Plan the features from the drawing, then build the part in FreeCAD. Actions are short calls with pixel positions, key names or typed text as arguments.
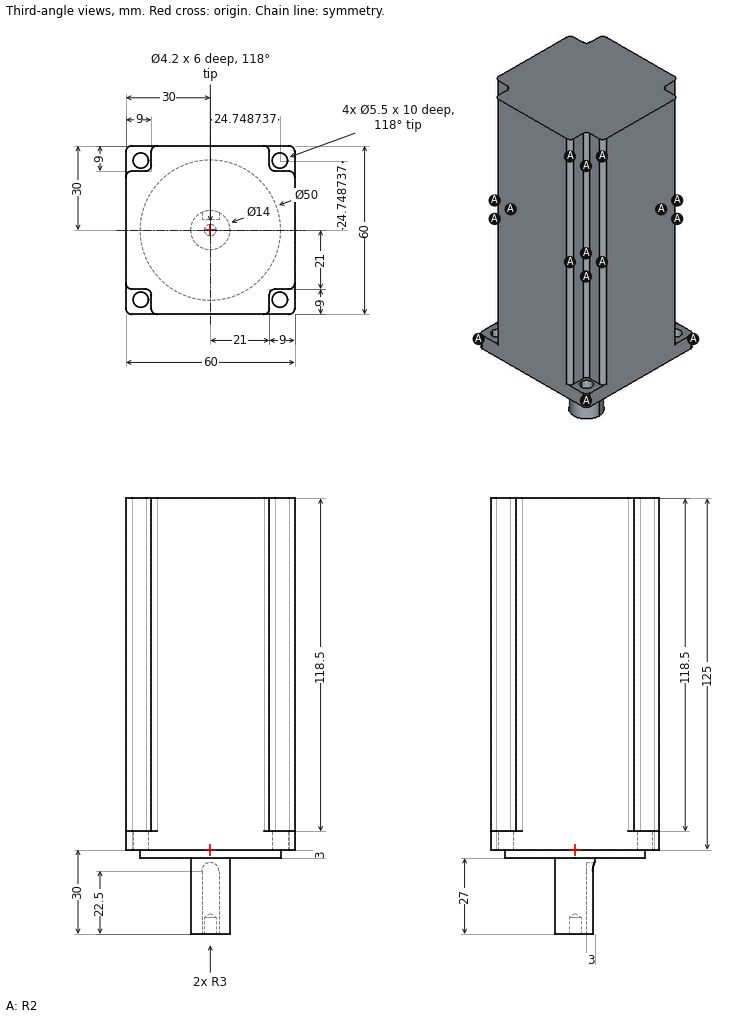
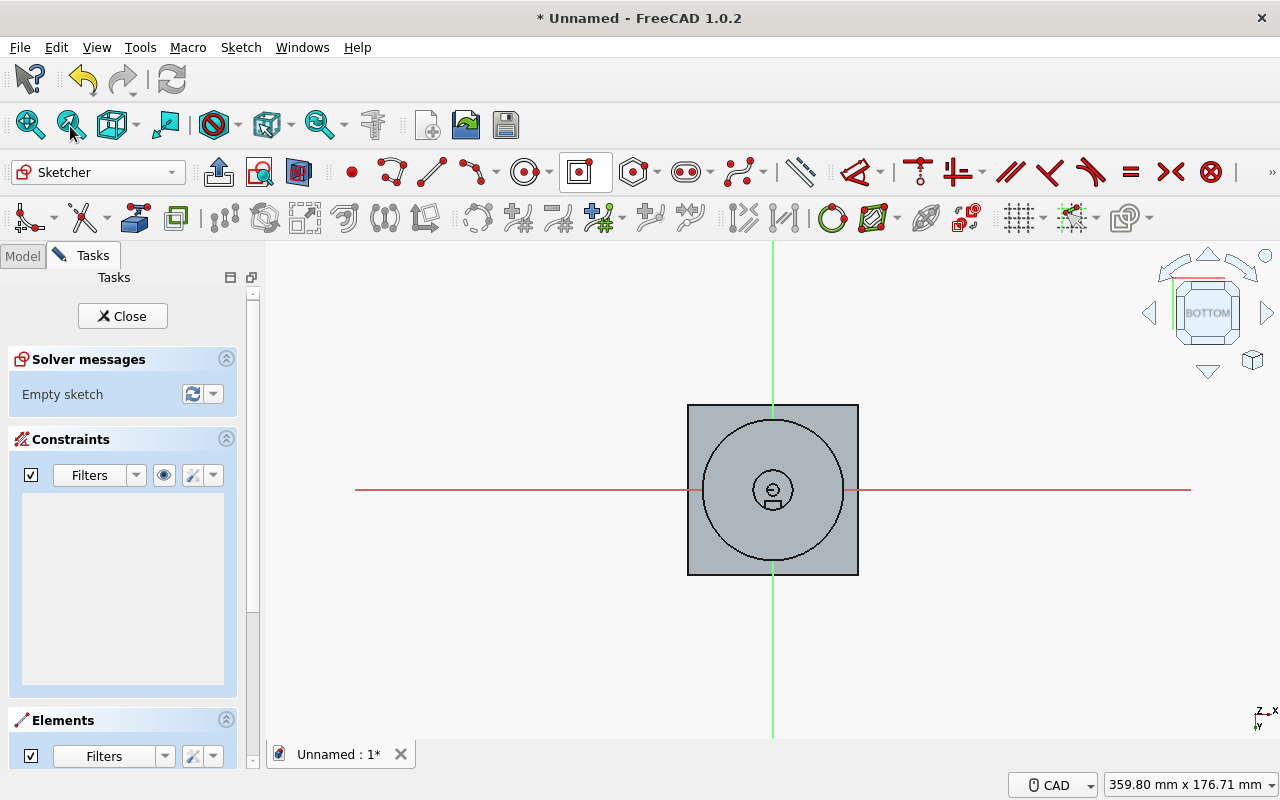
click(300, 172)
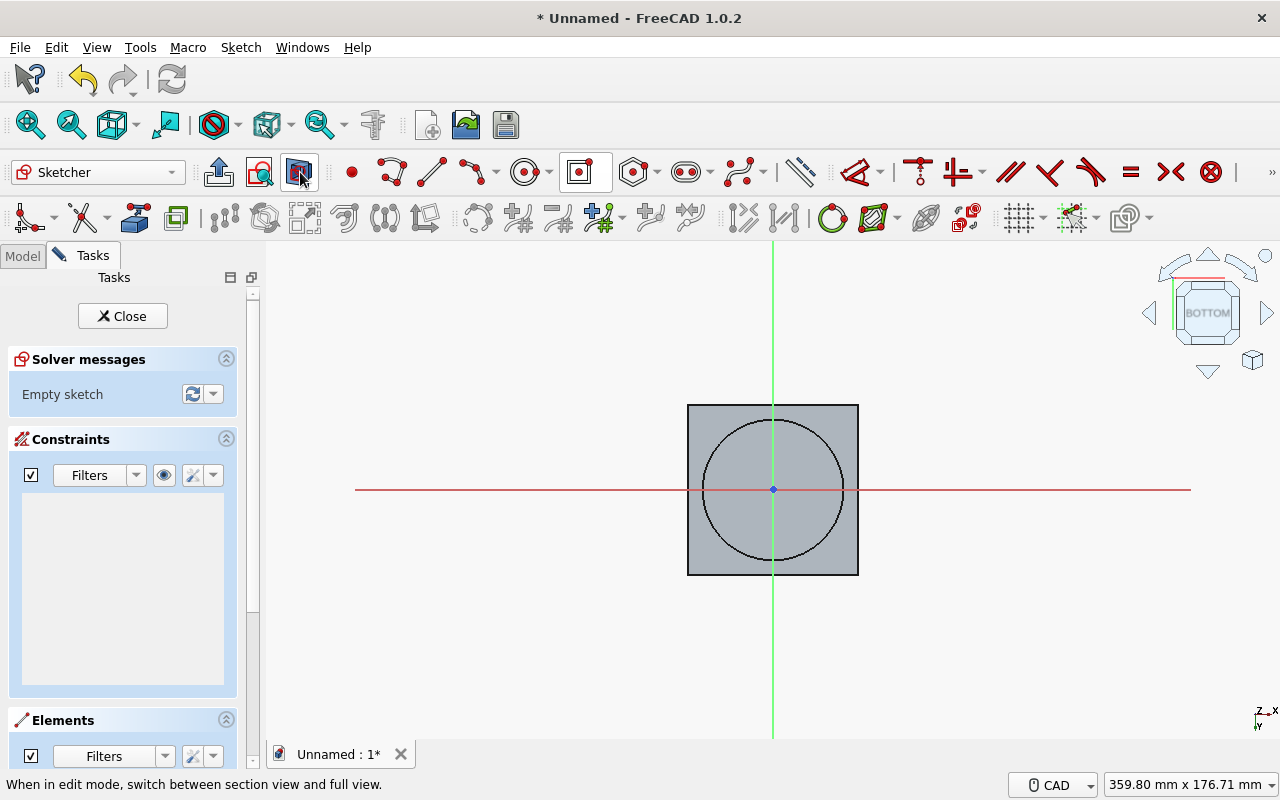
scroll(856, 490, up, 3)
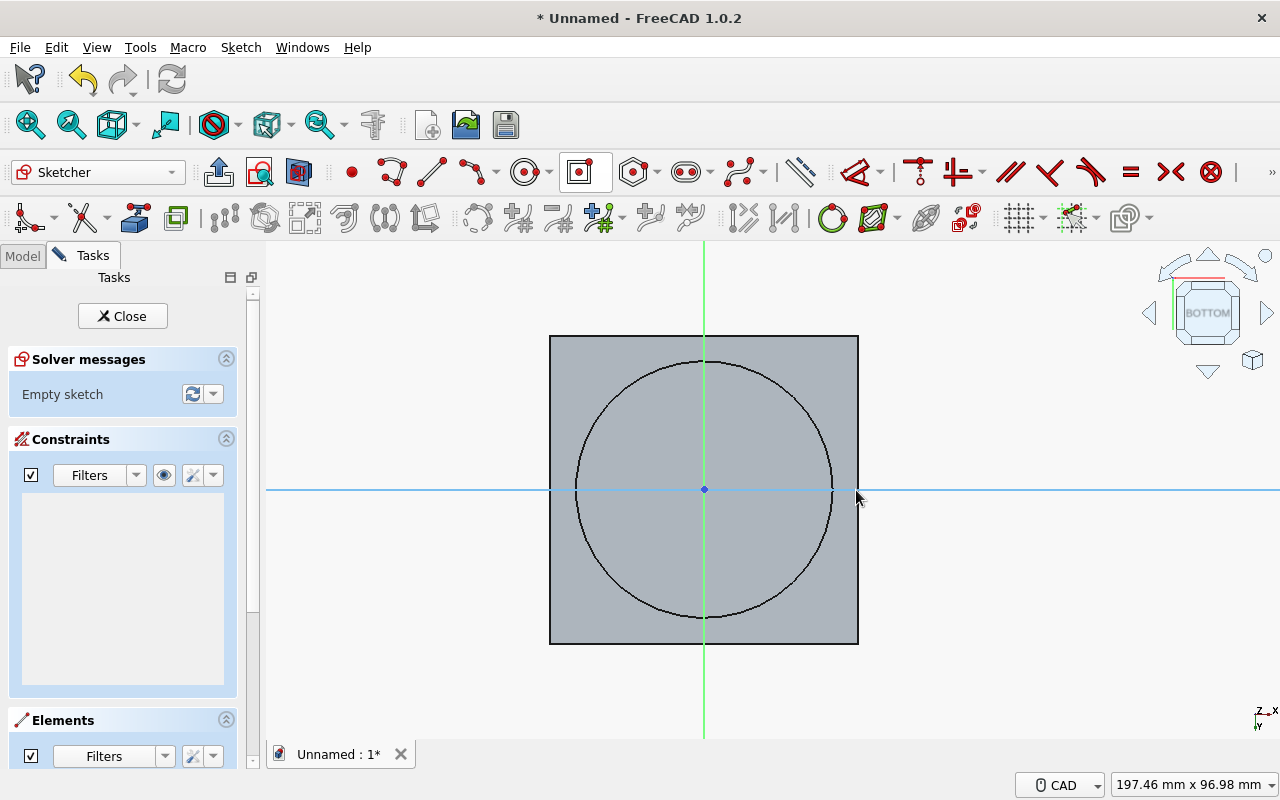
click(526, 172)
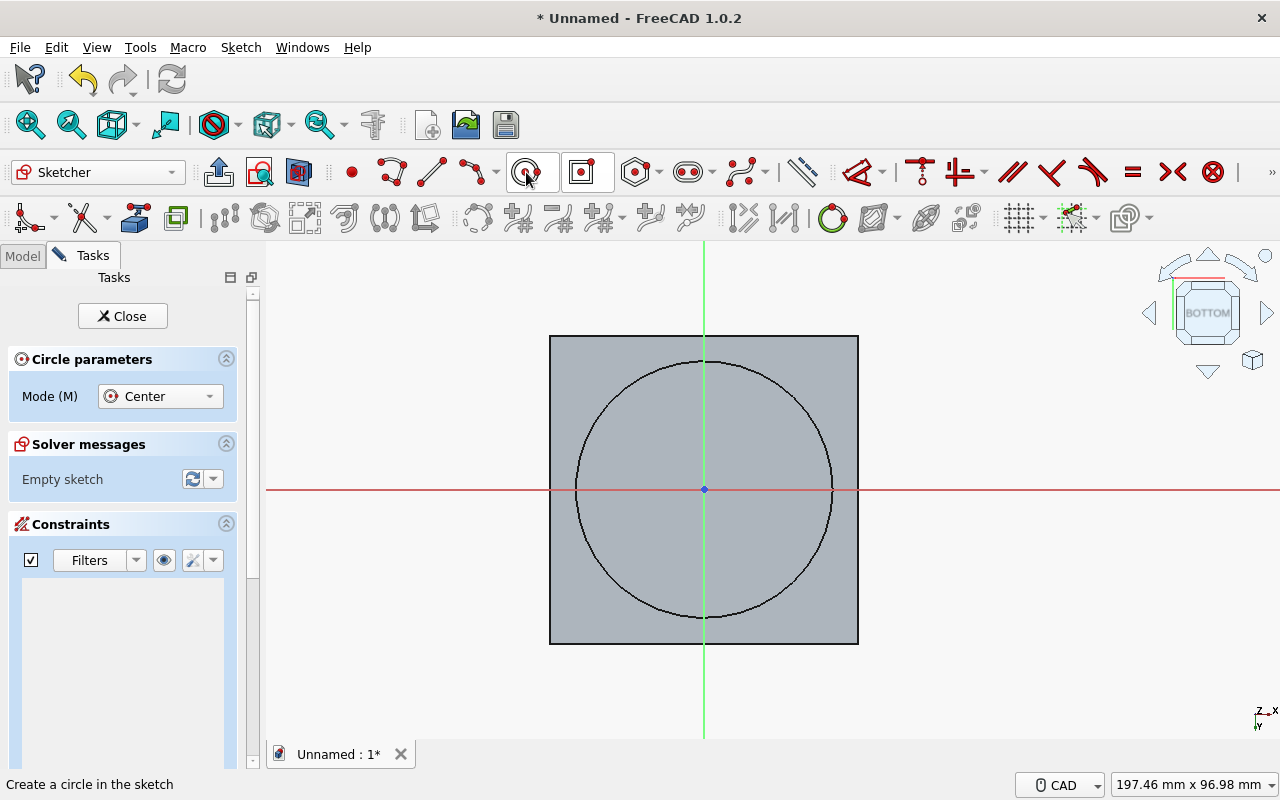
scroll(831, 617, up, 3)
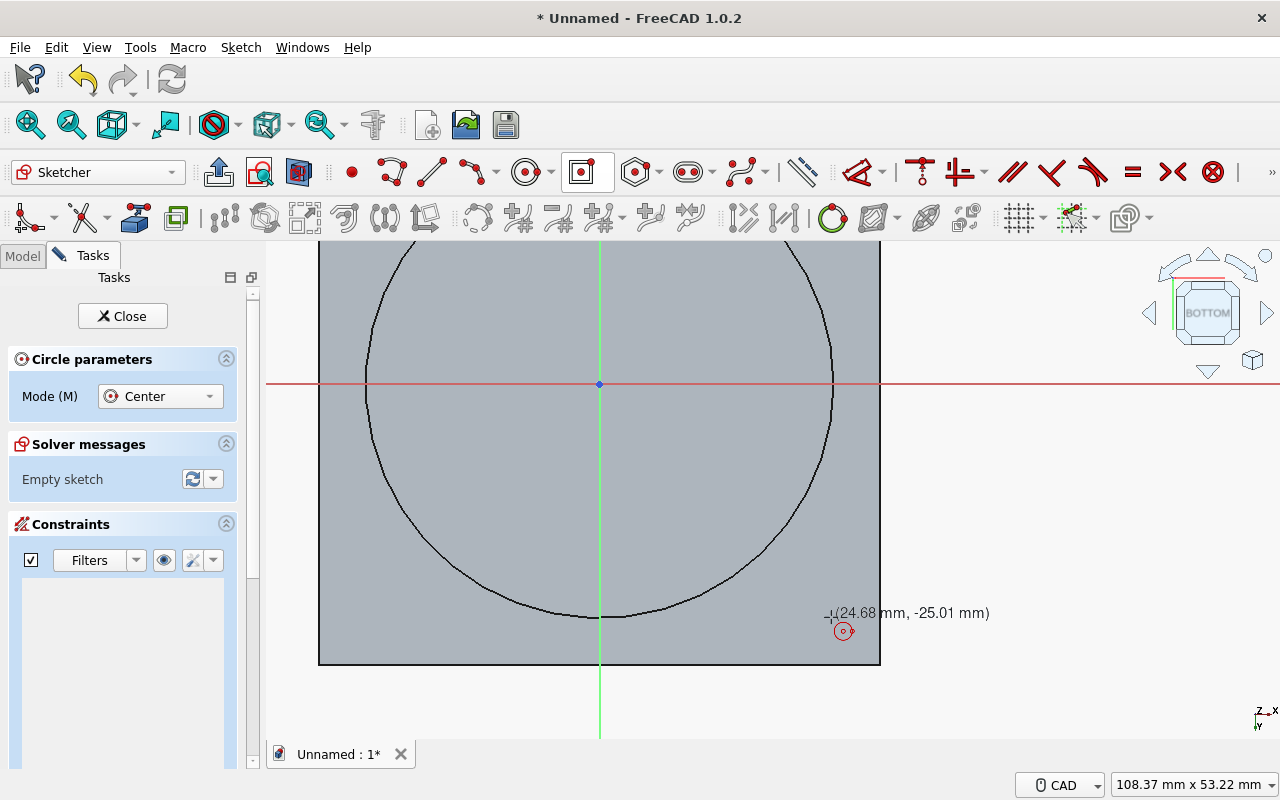
click(831, 616)
move(849, 598)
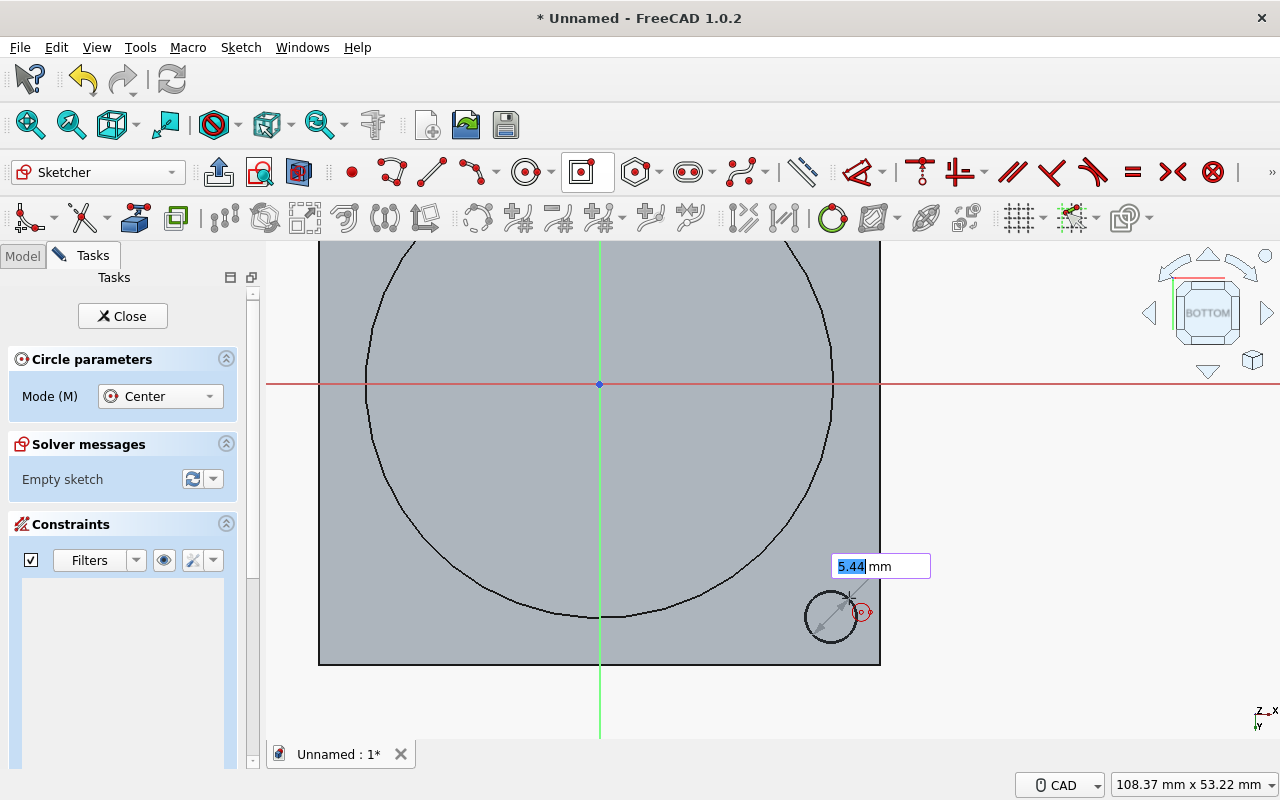
text(5.5)
key(Return)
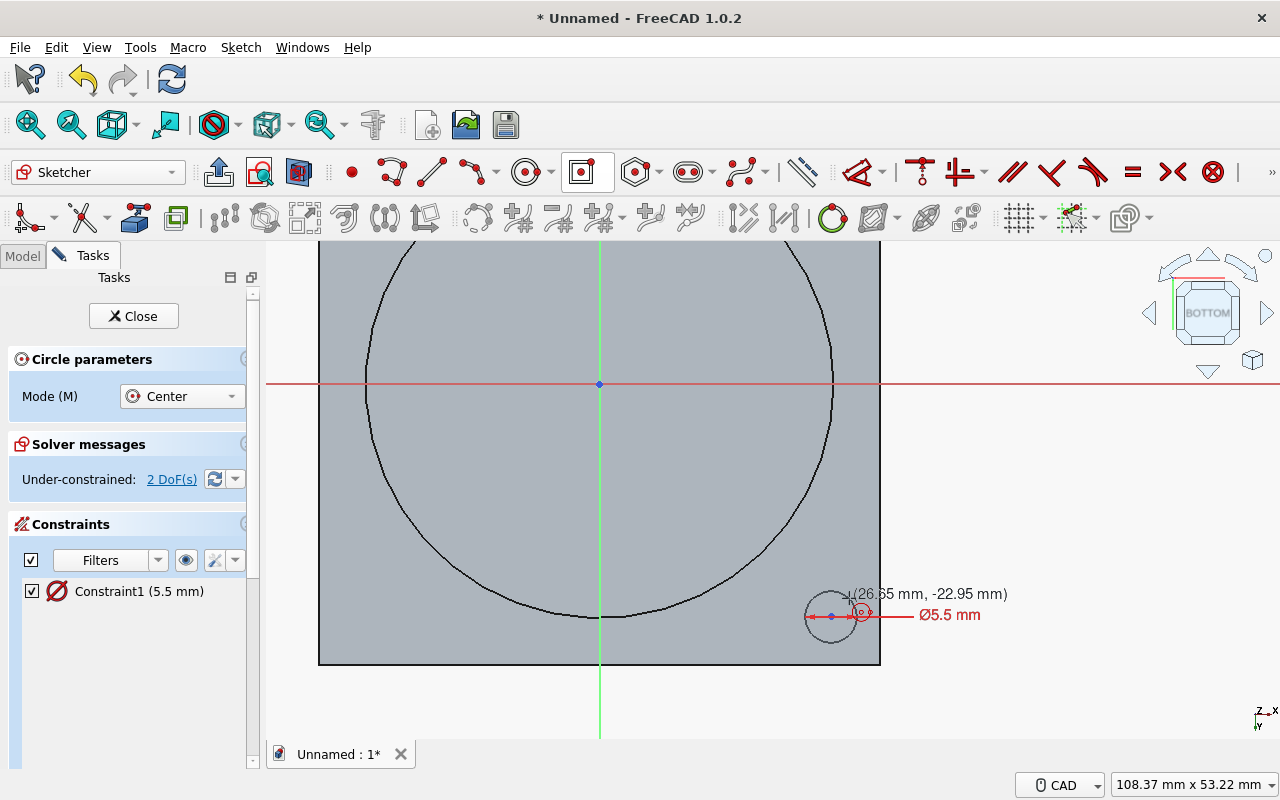
click(368, 616)
move(386, 598)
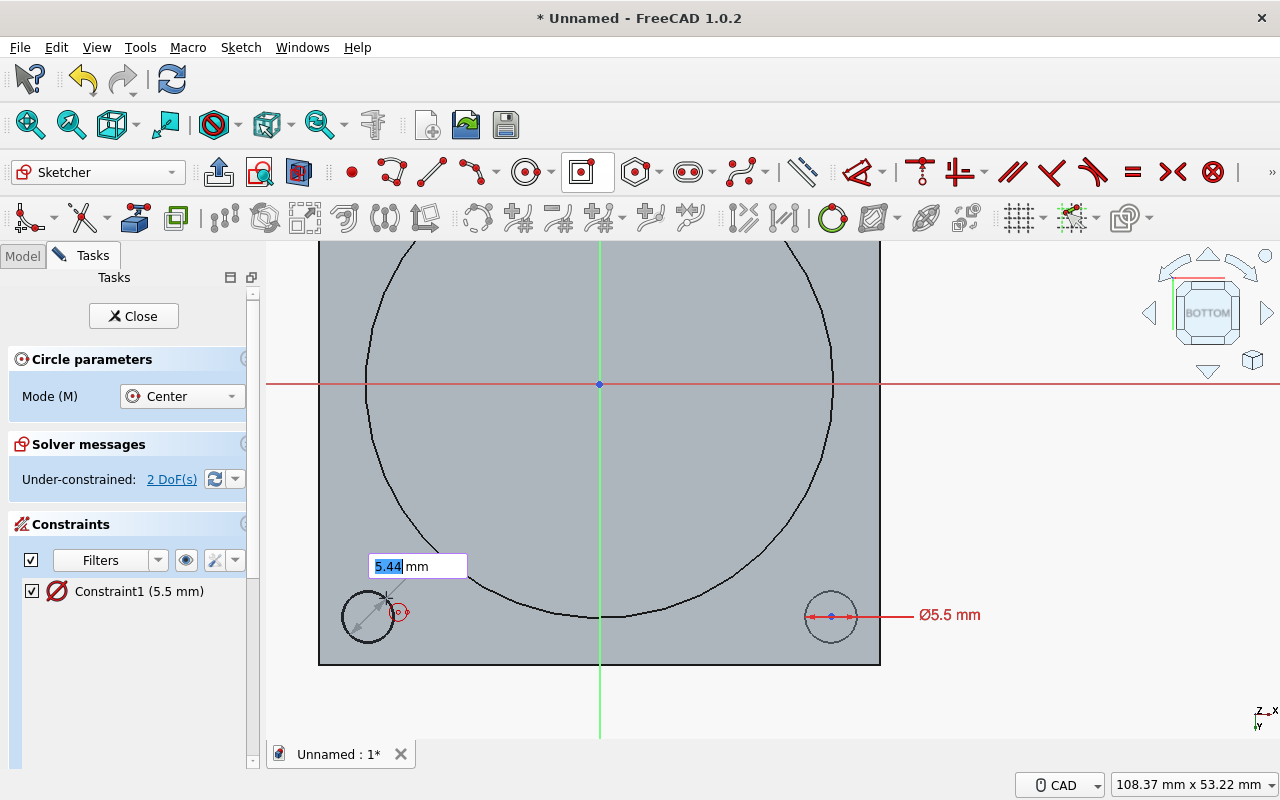
text(5.5)
key(Return)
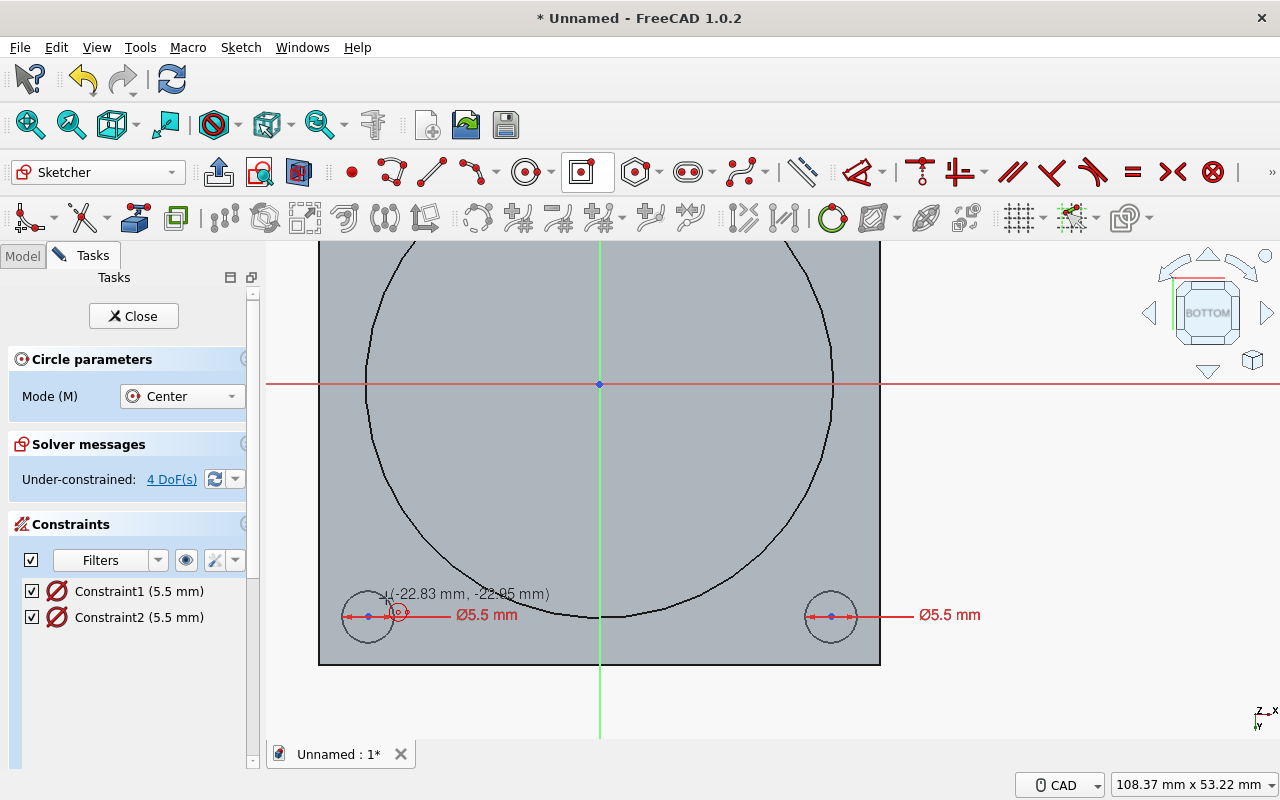
scroll(832, 619, down, 3)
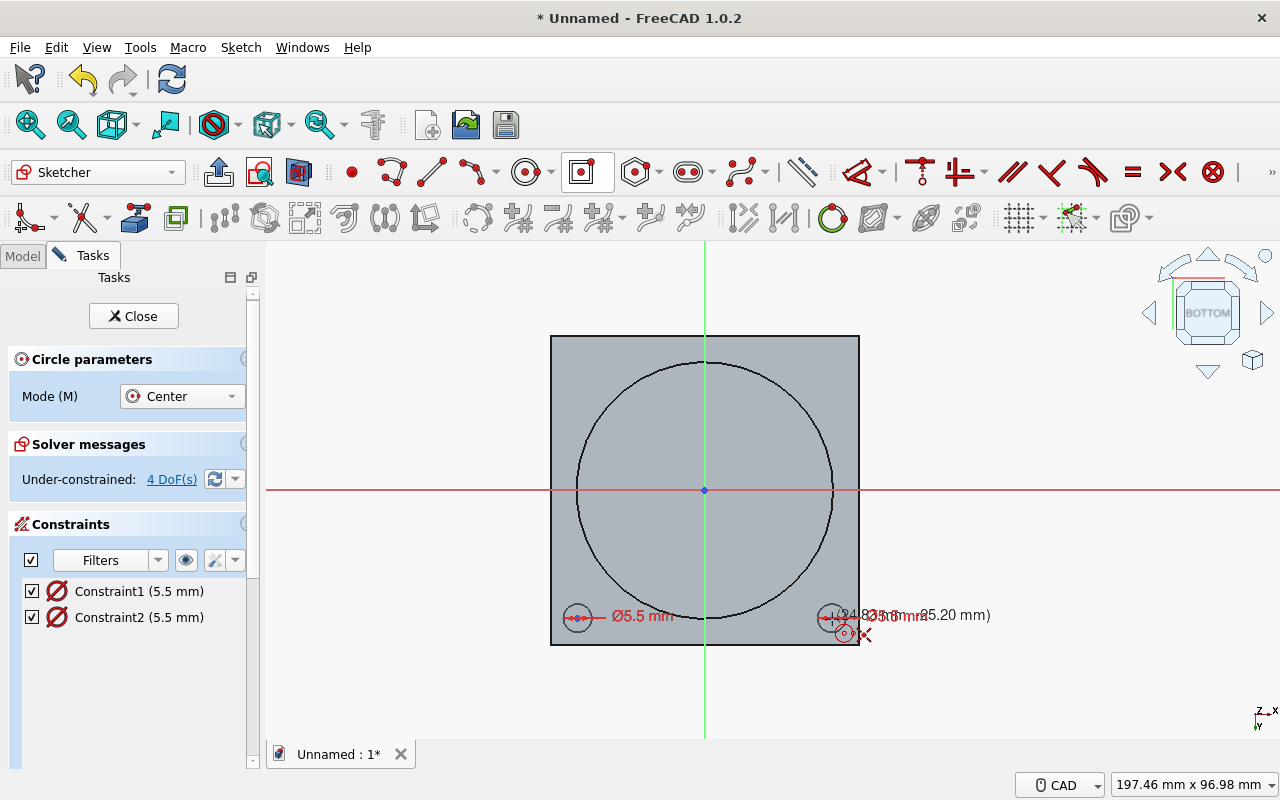
scroll(578, 363, up, 3)